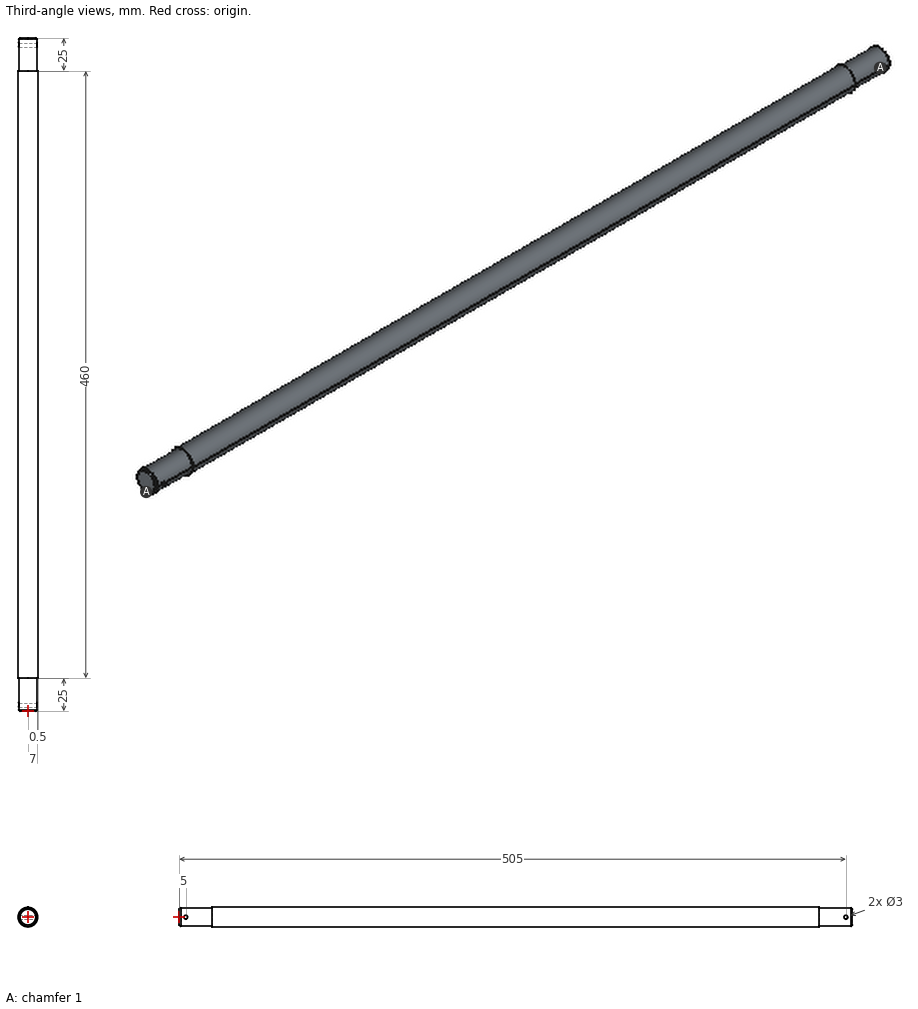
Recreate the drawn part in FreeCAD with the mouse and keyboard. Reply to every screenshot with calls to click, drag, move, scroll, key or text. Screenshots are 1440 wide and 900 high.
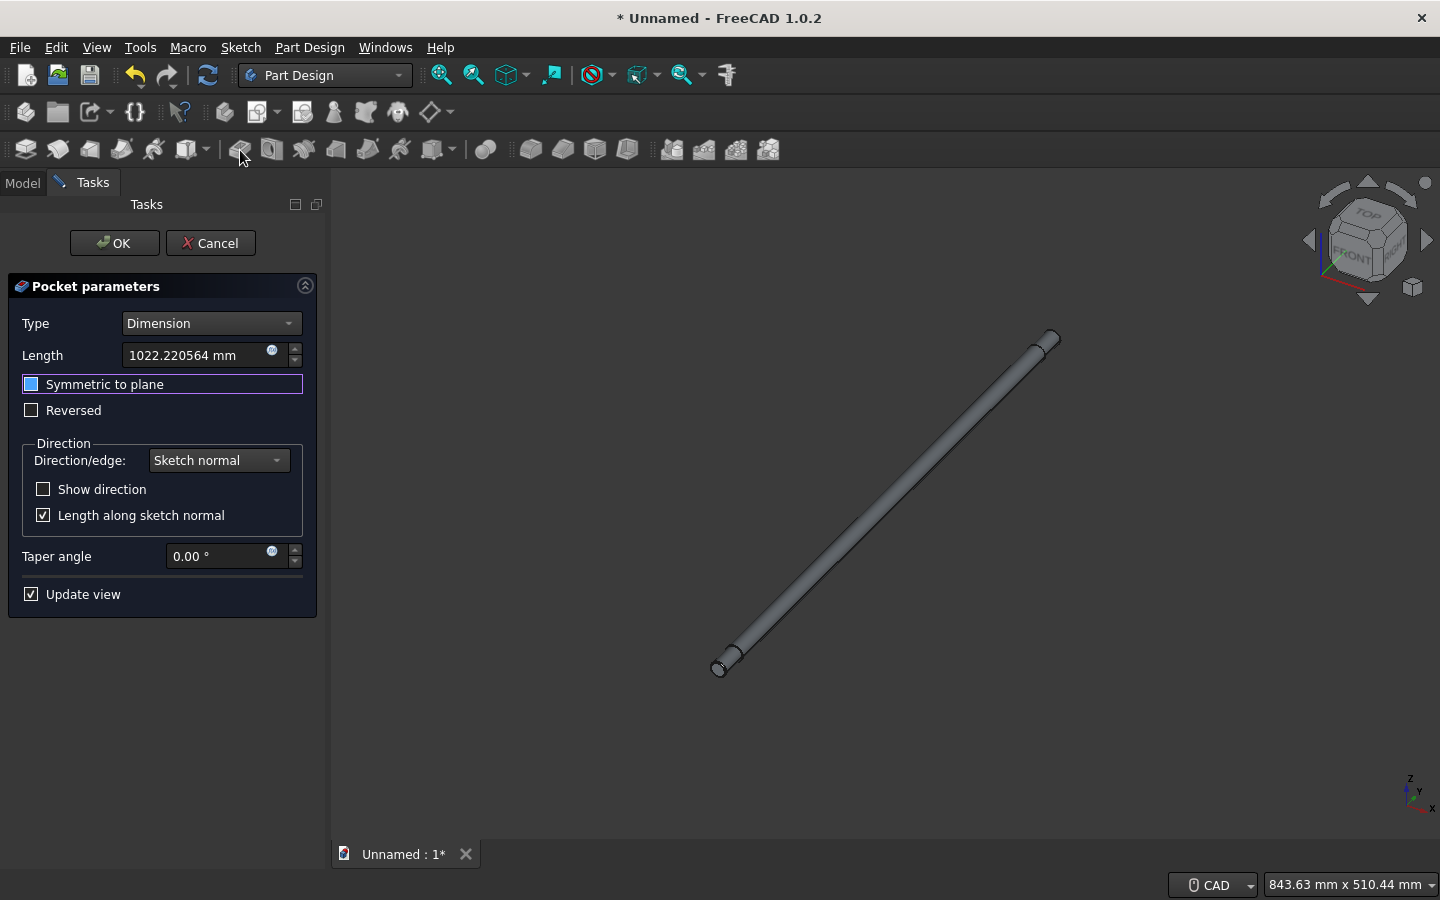
click(30, 384)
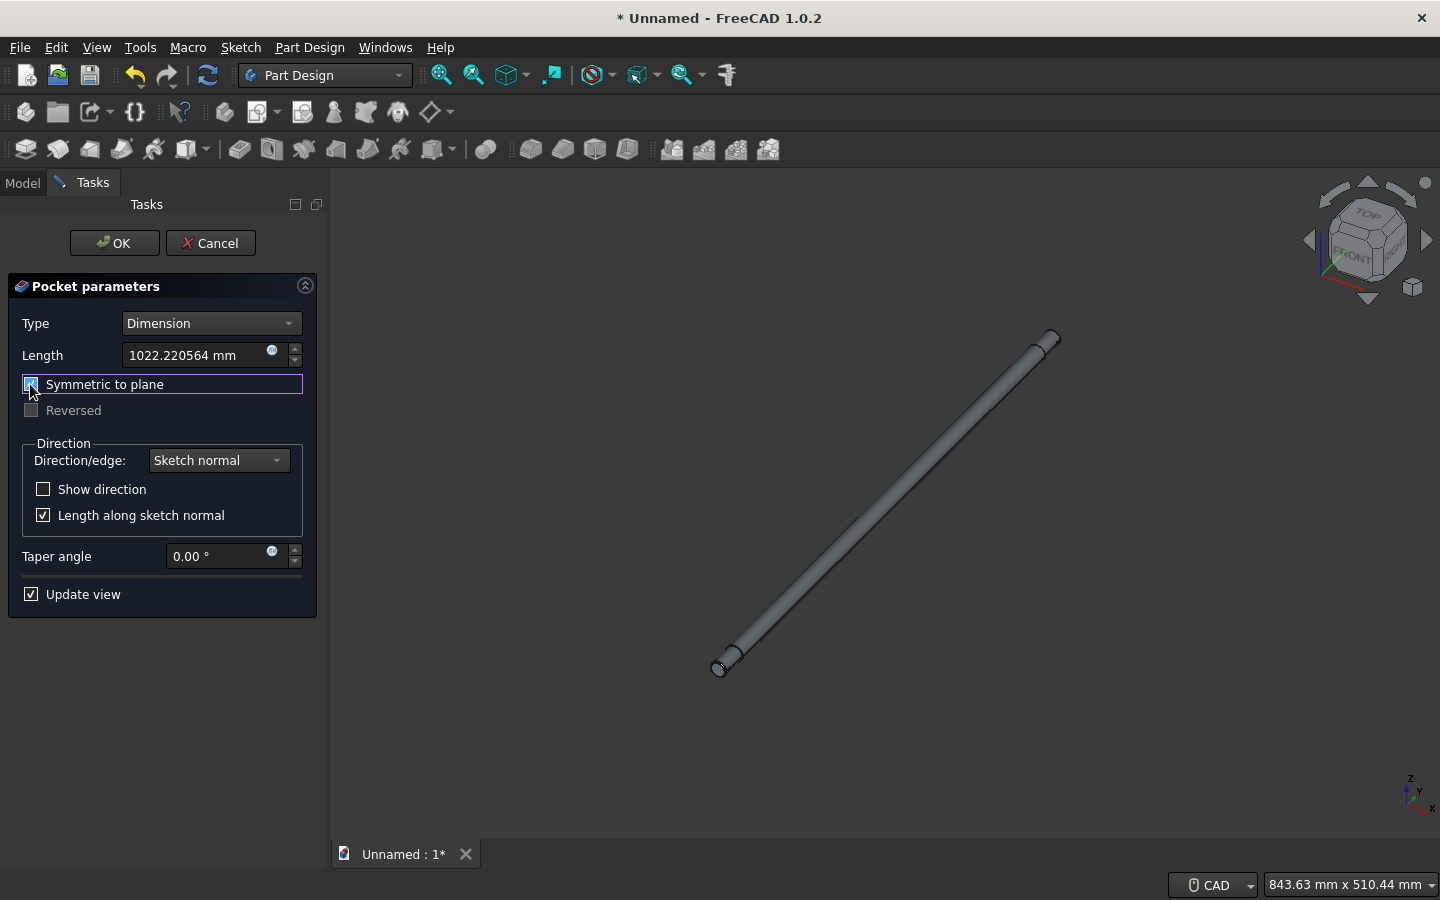
click(115, 243)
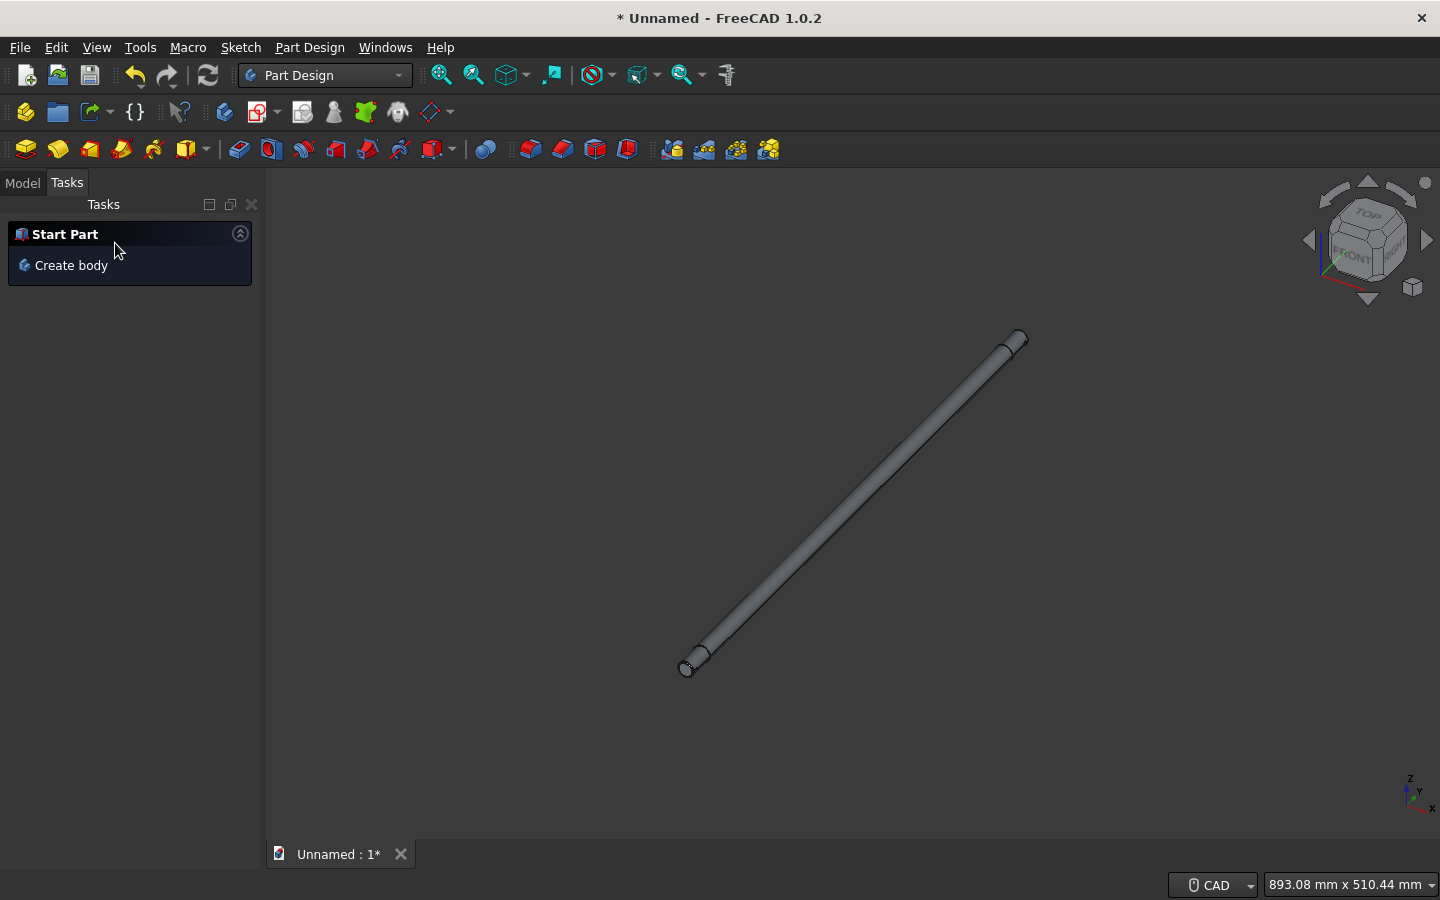
key(0)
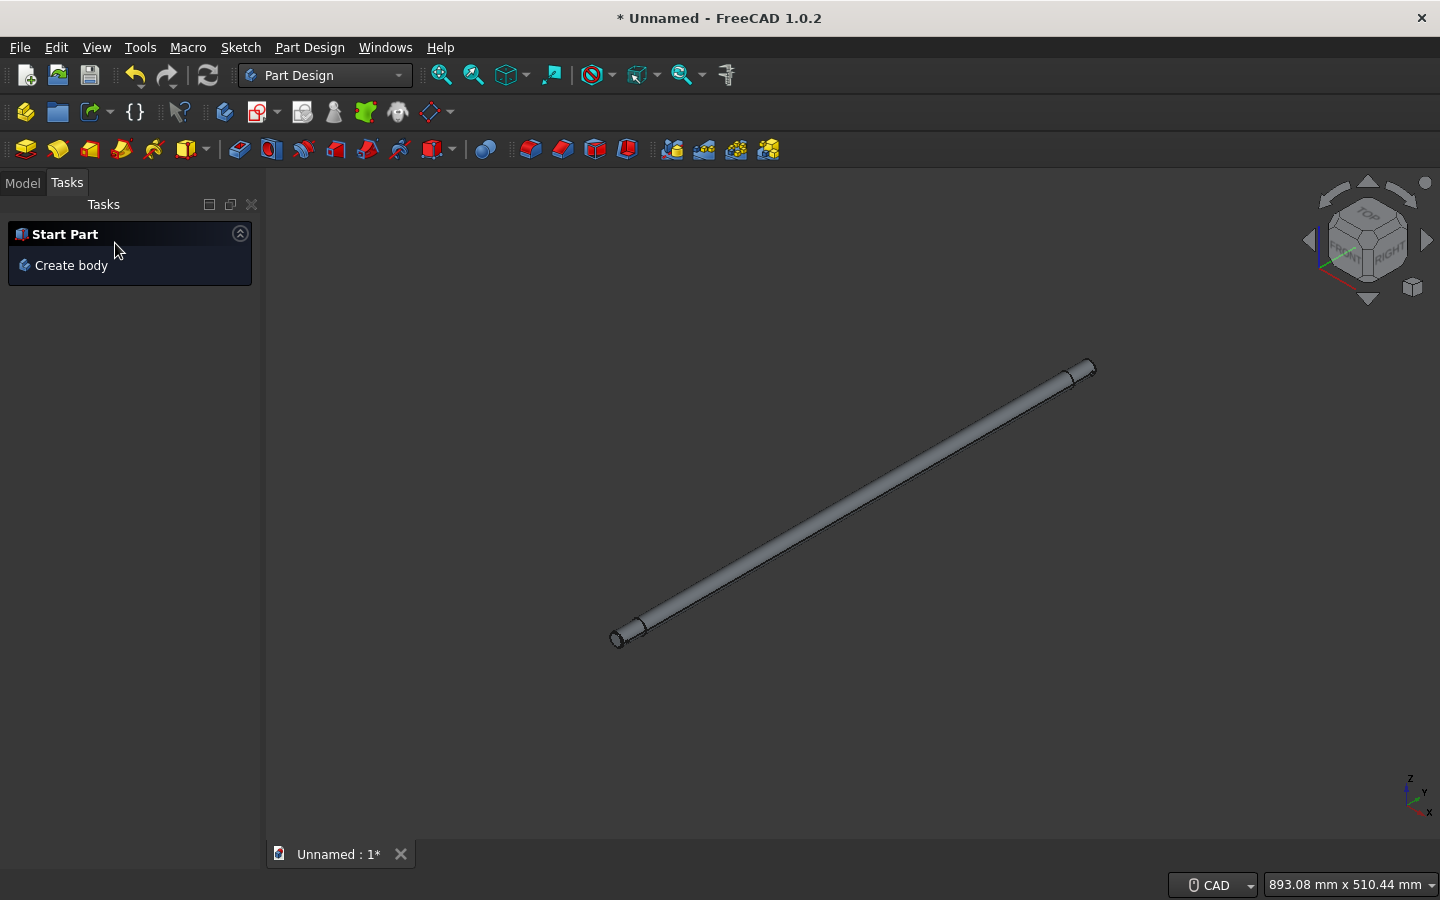
click(442, 76)